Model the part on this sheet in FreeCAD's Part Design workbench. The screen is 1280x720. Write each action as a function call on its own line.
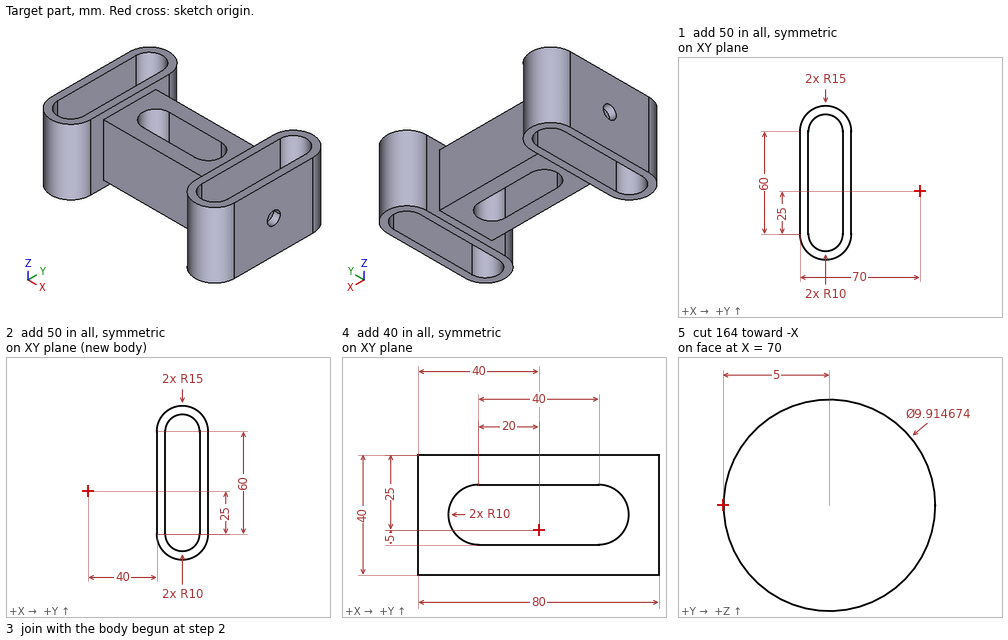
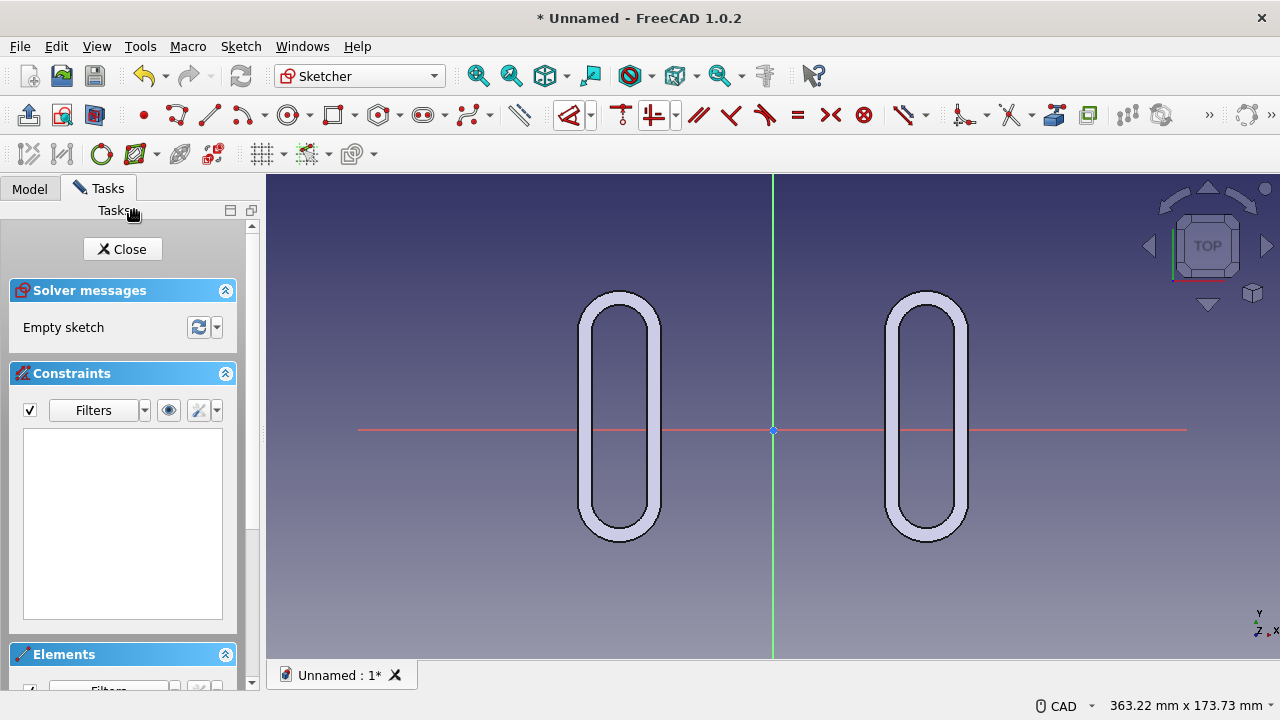
click(95, 116)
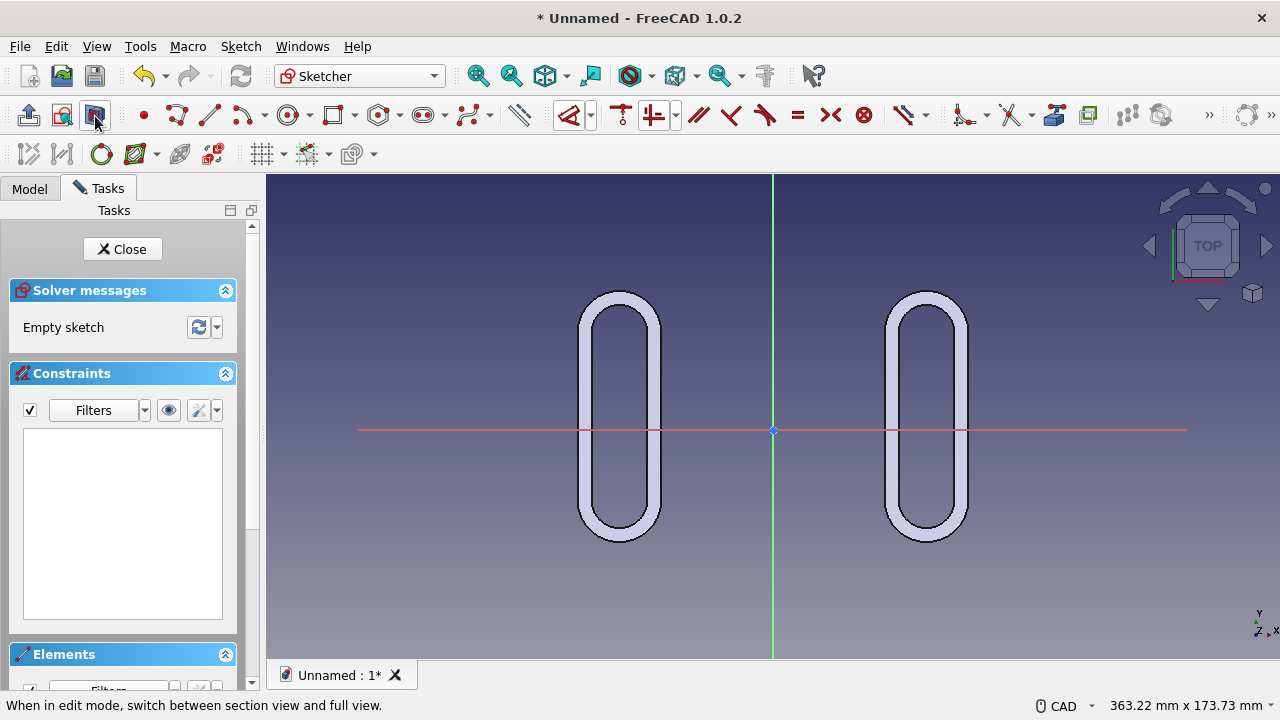
scroll(813, 416, up, 5)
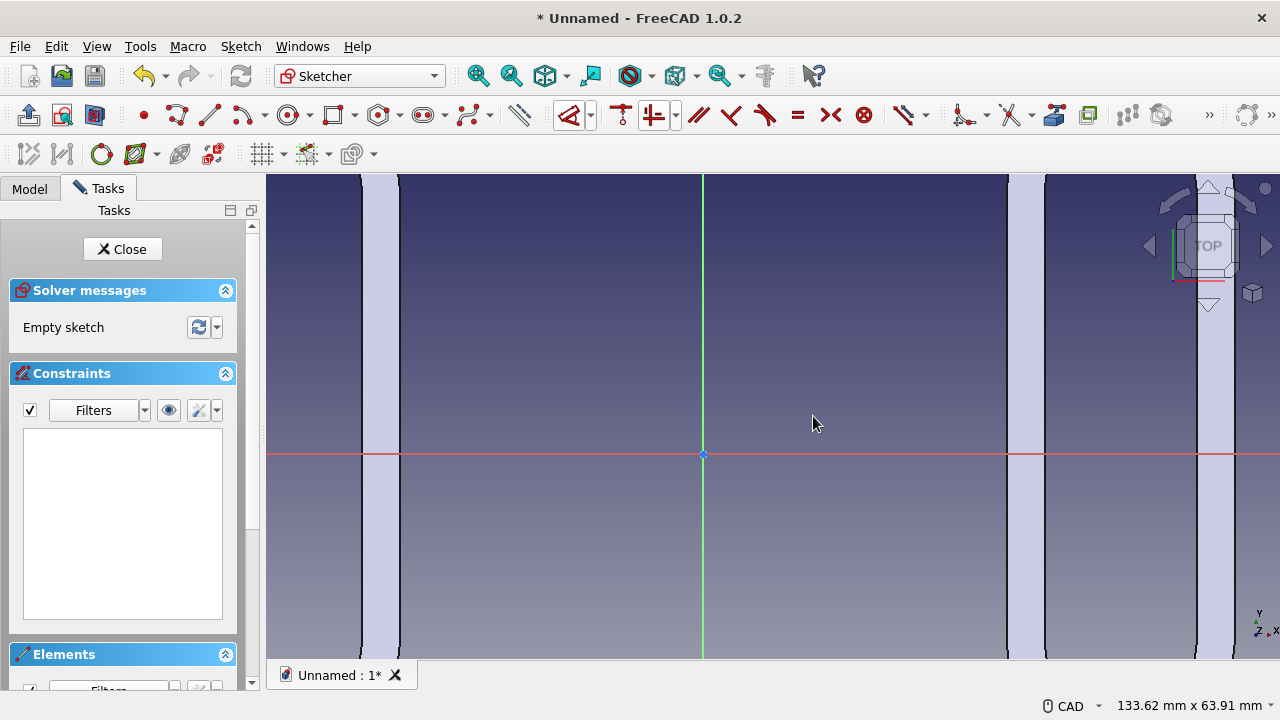
click(332, 116)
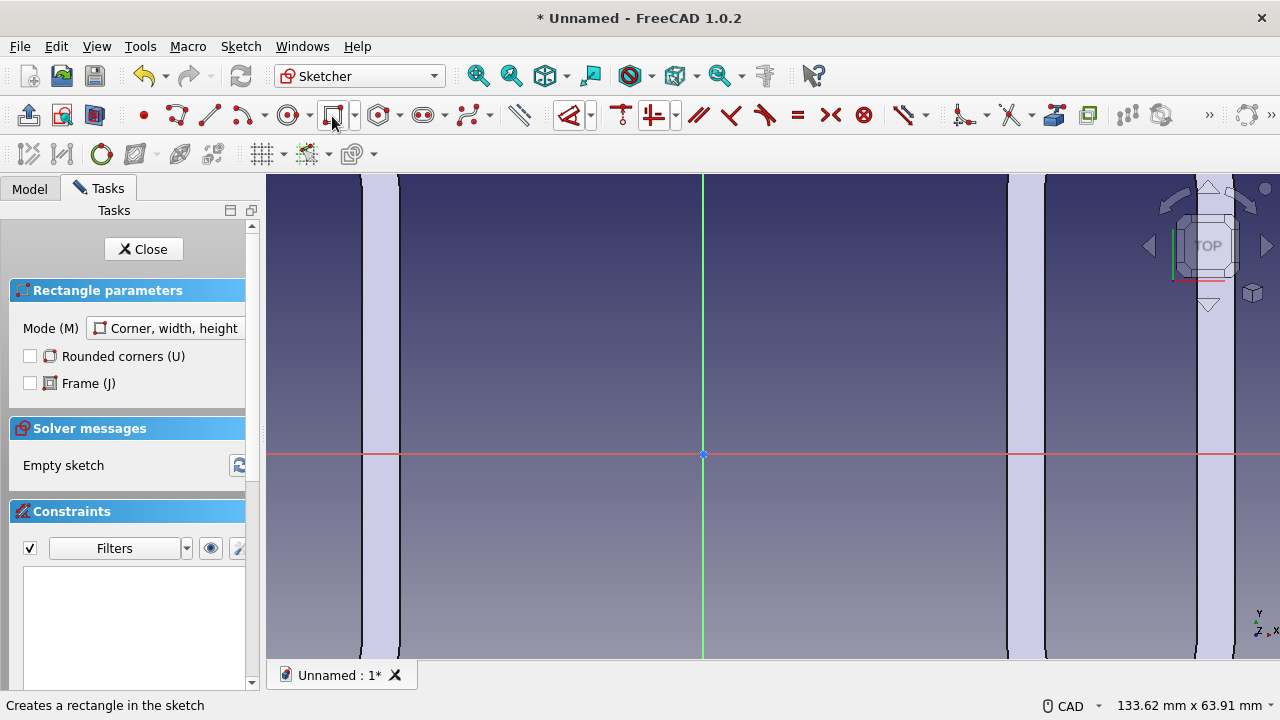
click(400, 265)
click(1007, 568)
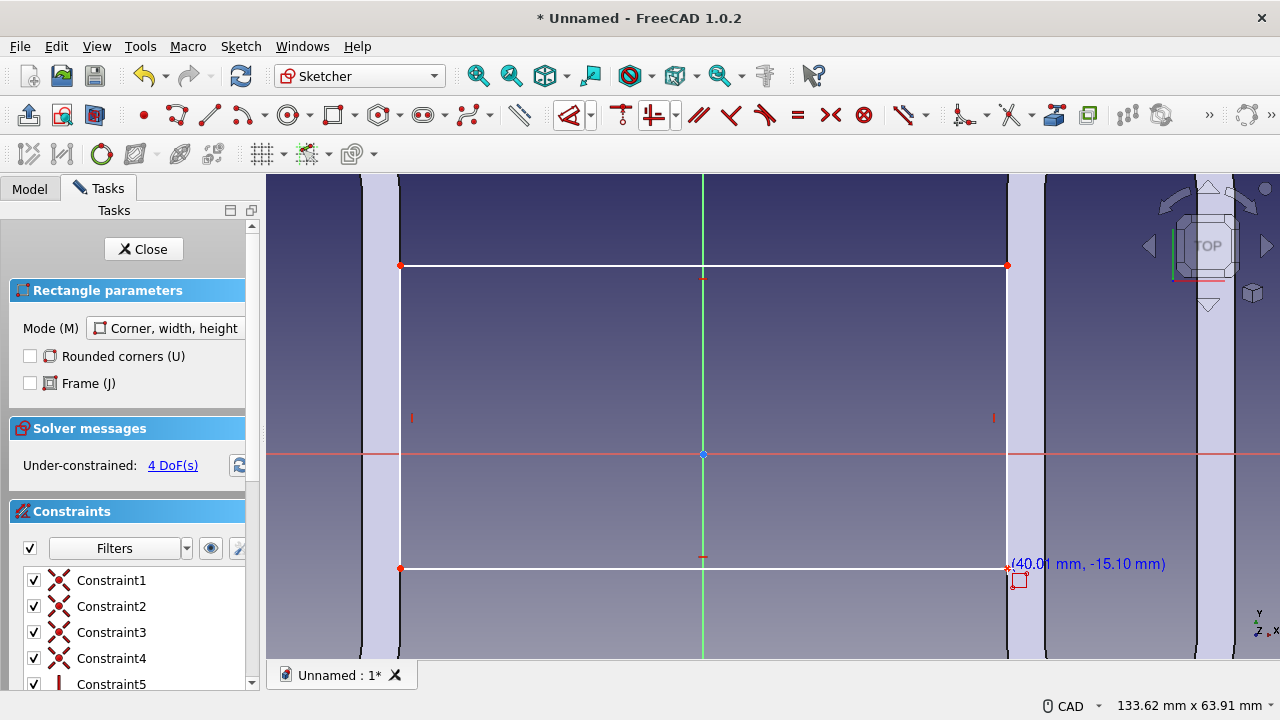
click(422, 116)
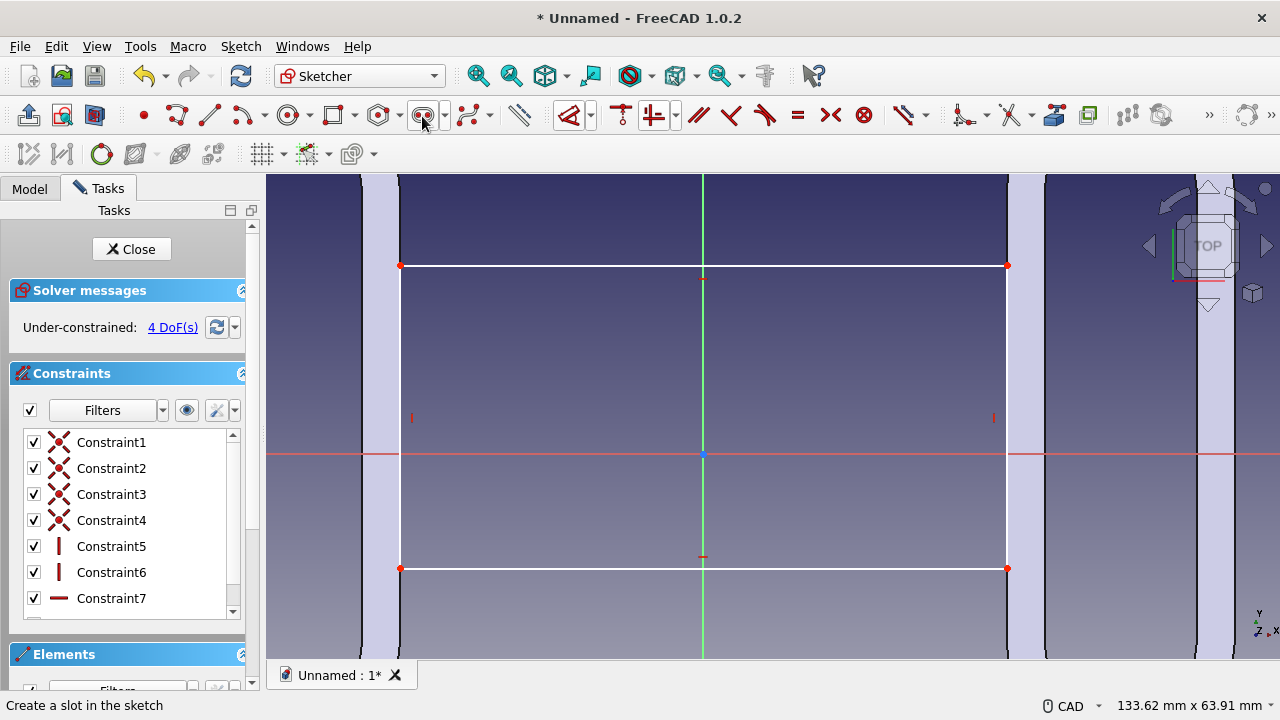
click(552, 416)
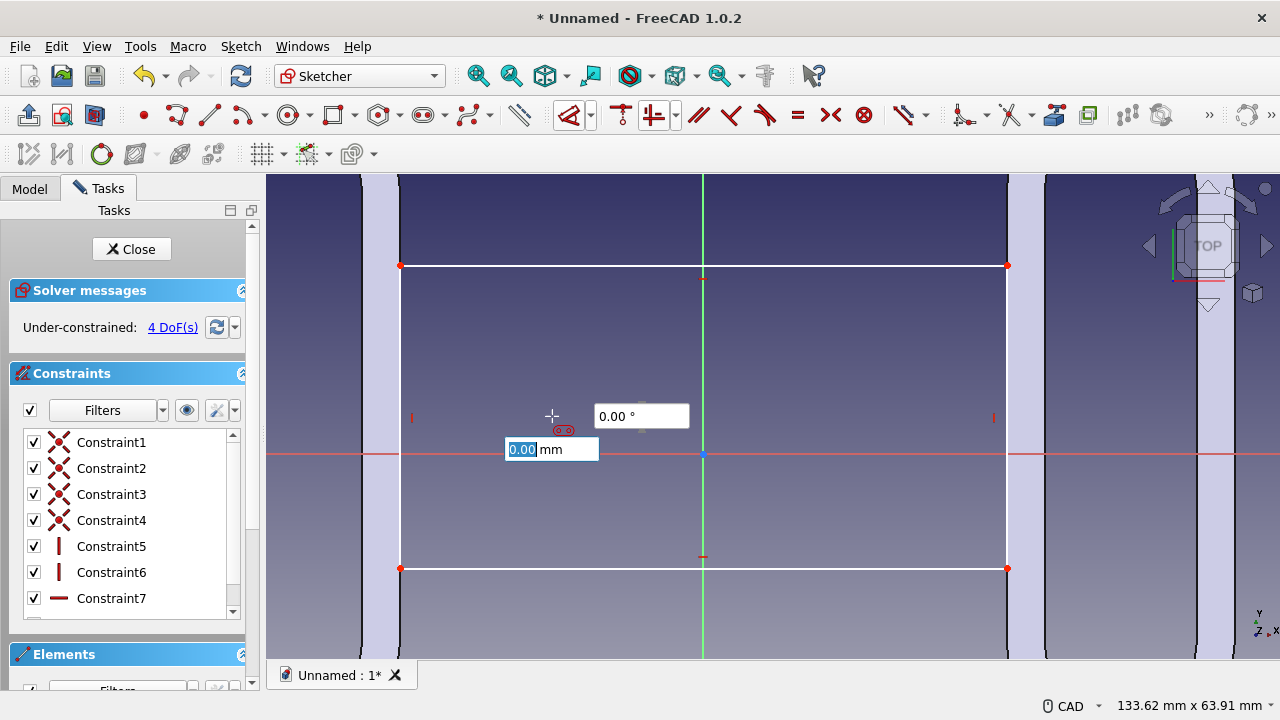
click(855, 416)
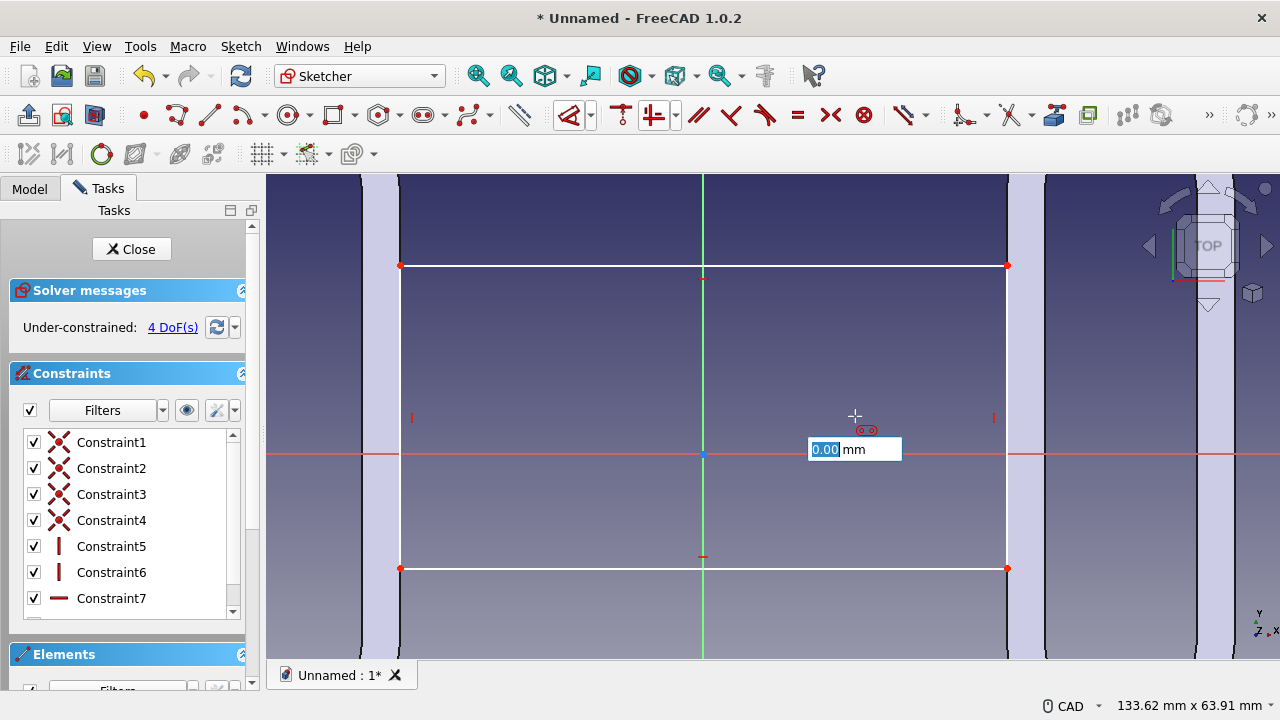
click(658, 341)
key(Escape)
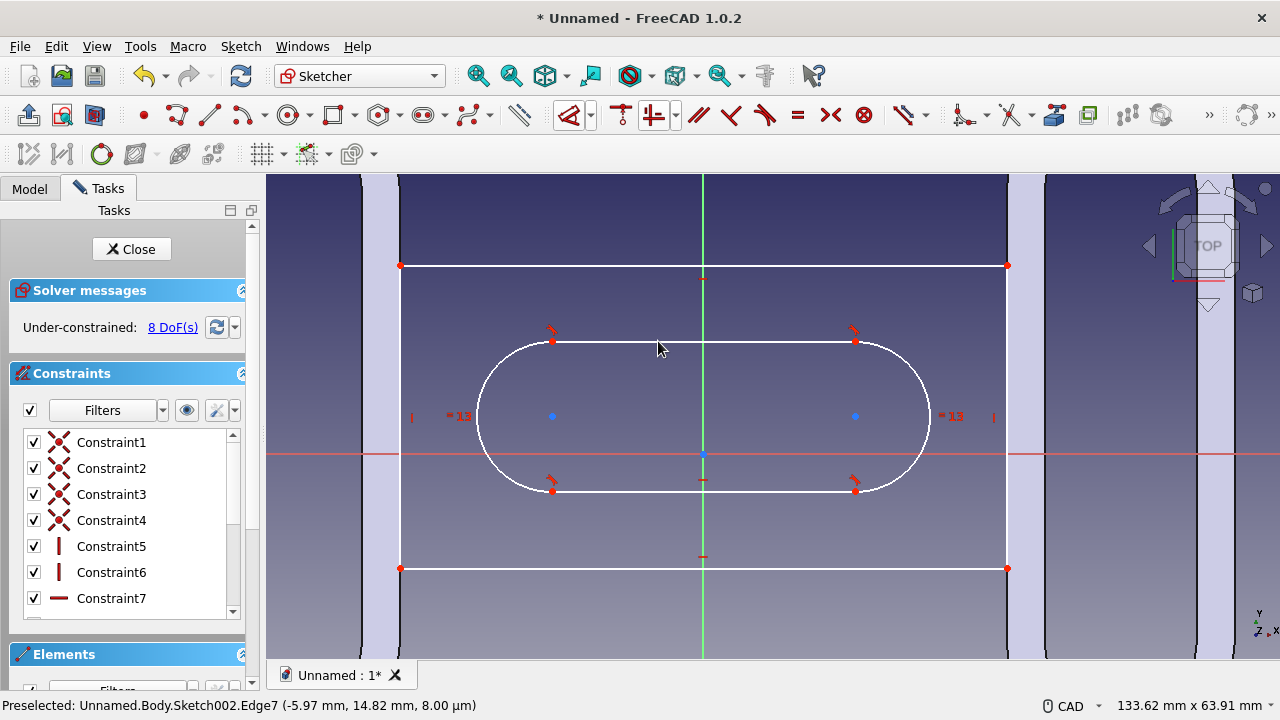
click(491, 373)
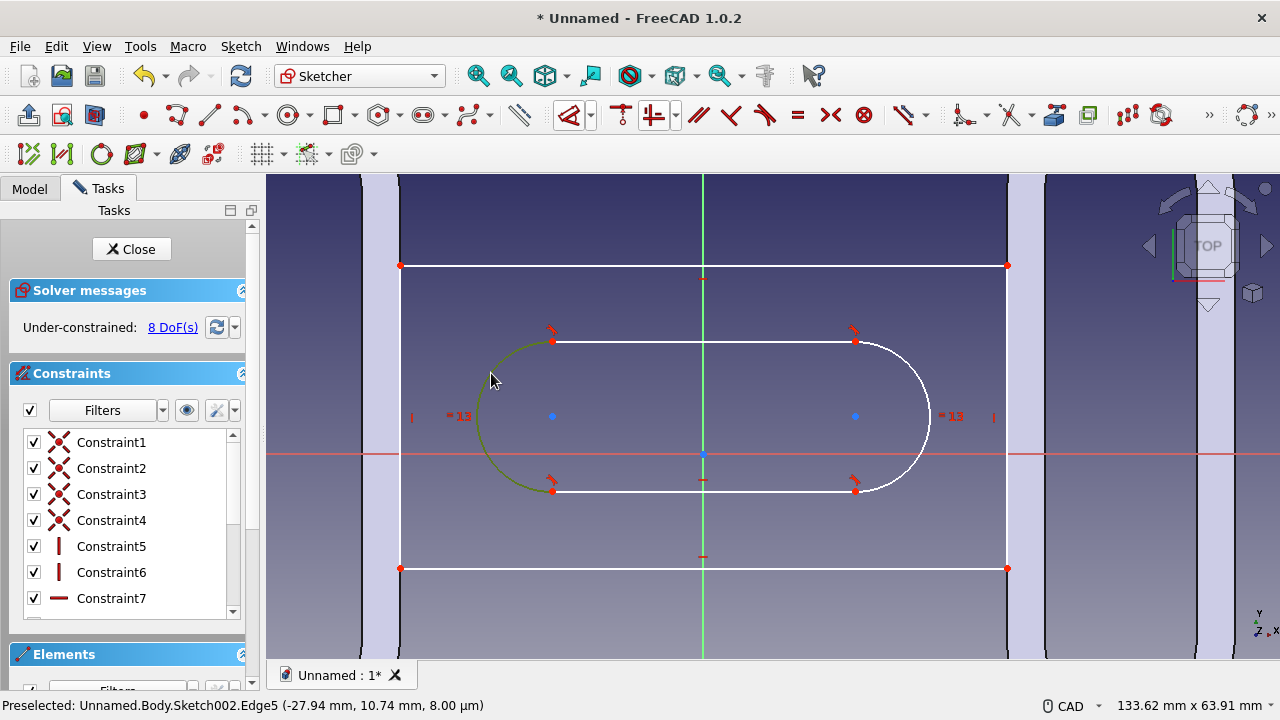
key(k)
key(r)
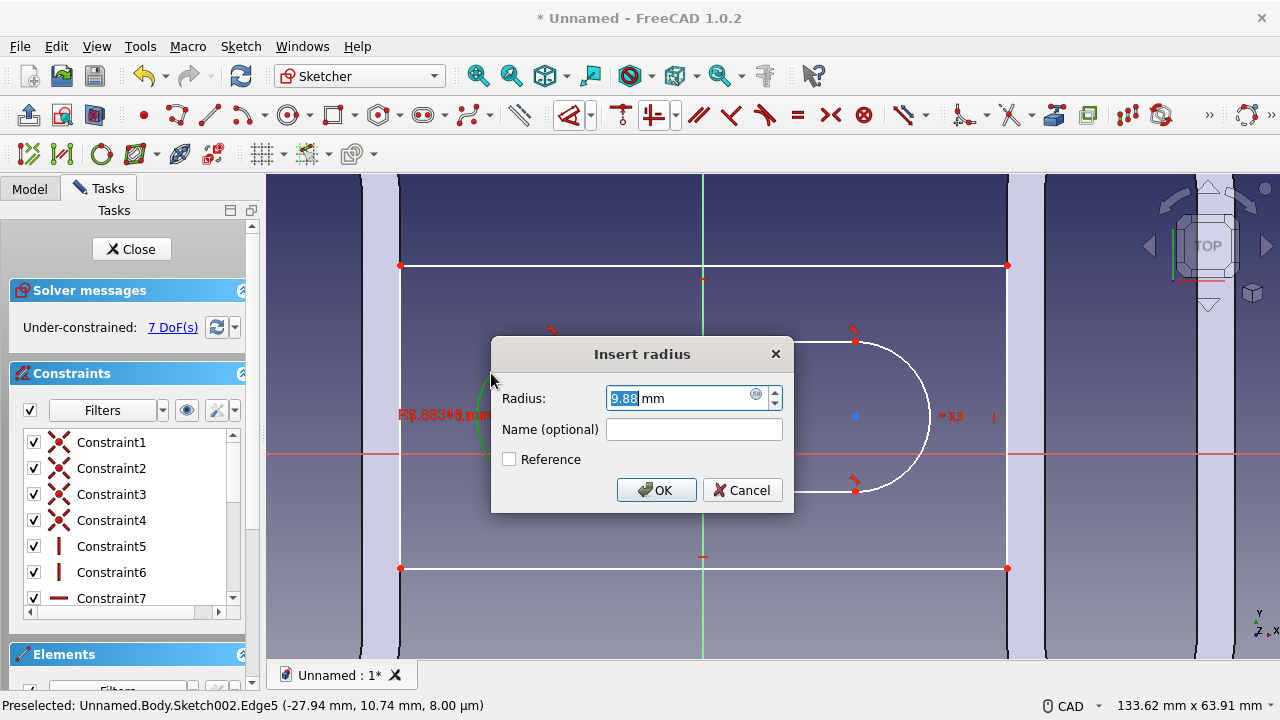
text(10)
key(Return)